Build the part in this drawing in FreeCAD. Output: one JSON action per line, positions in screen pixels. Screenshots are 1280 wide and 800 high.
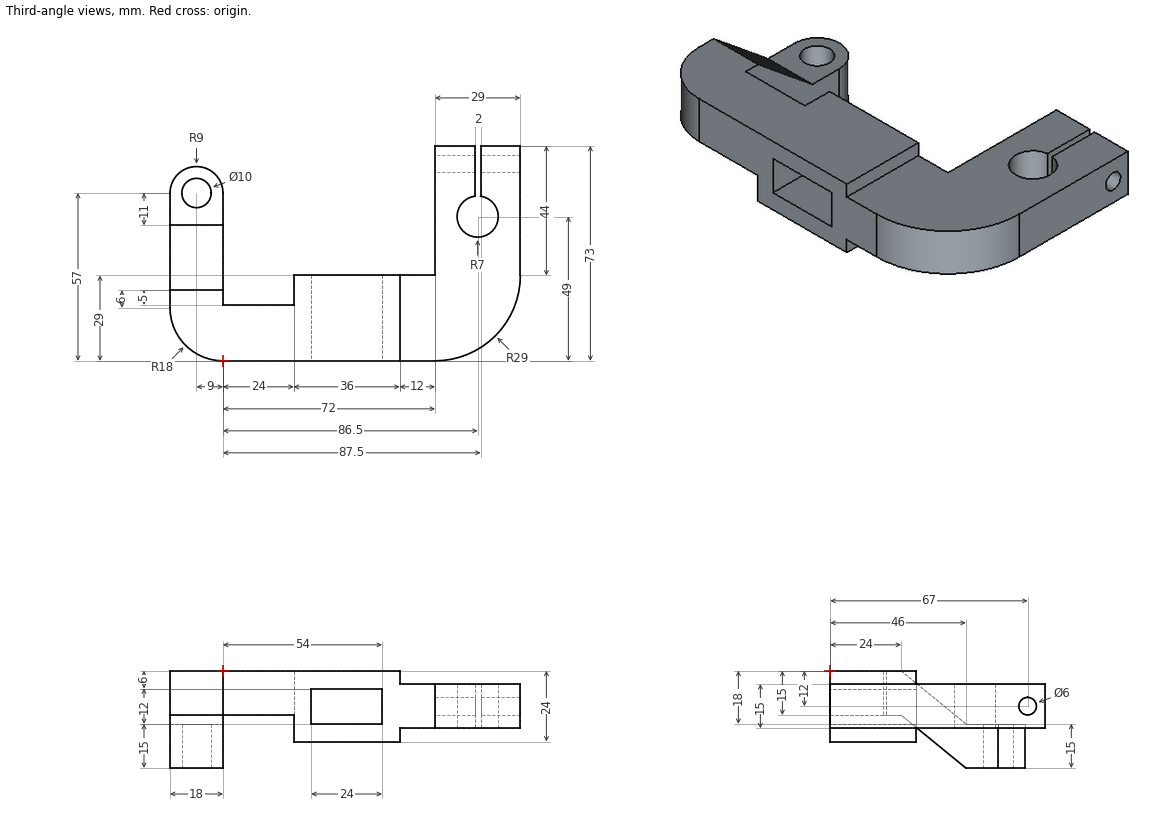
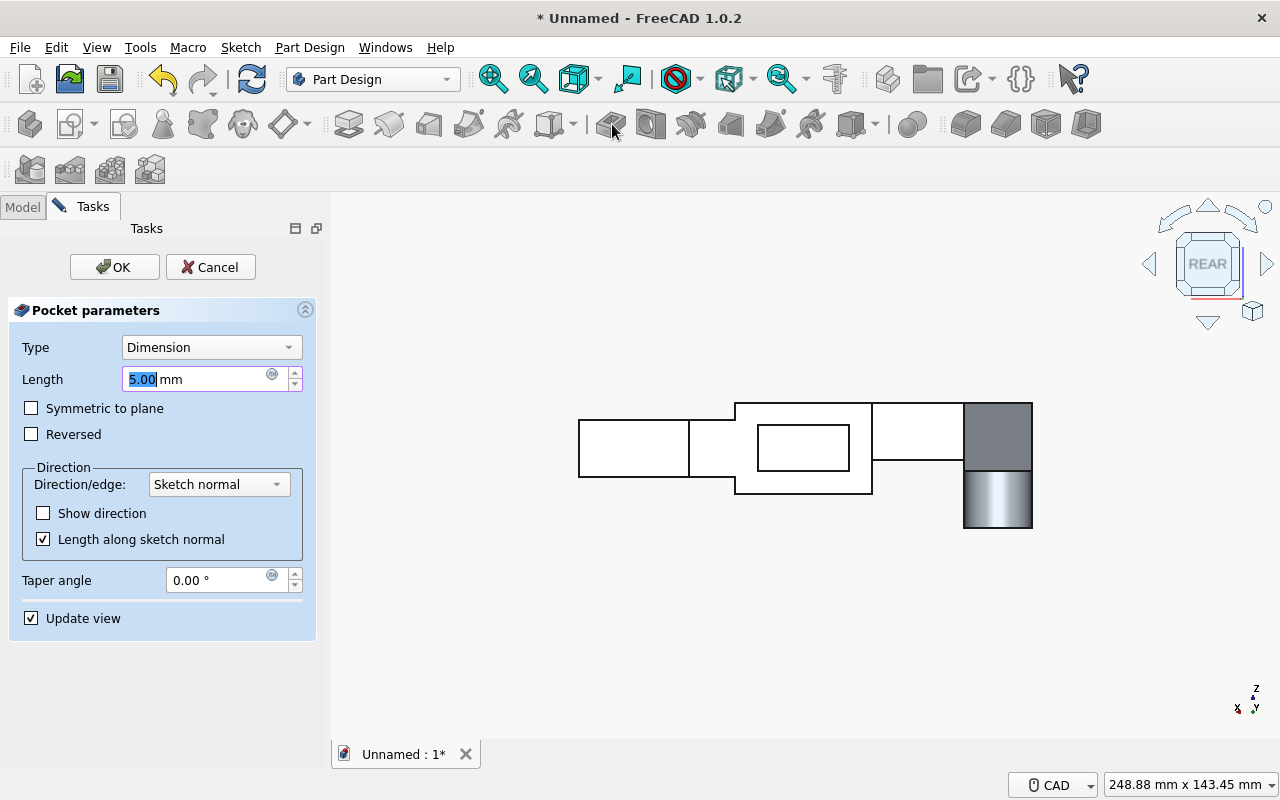
{"action": "left_click", "coordinate": [212, 348]}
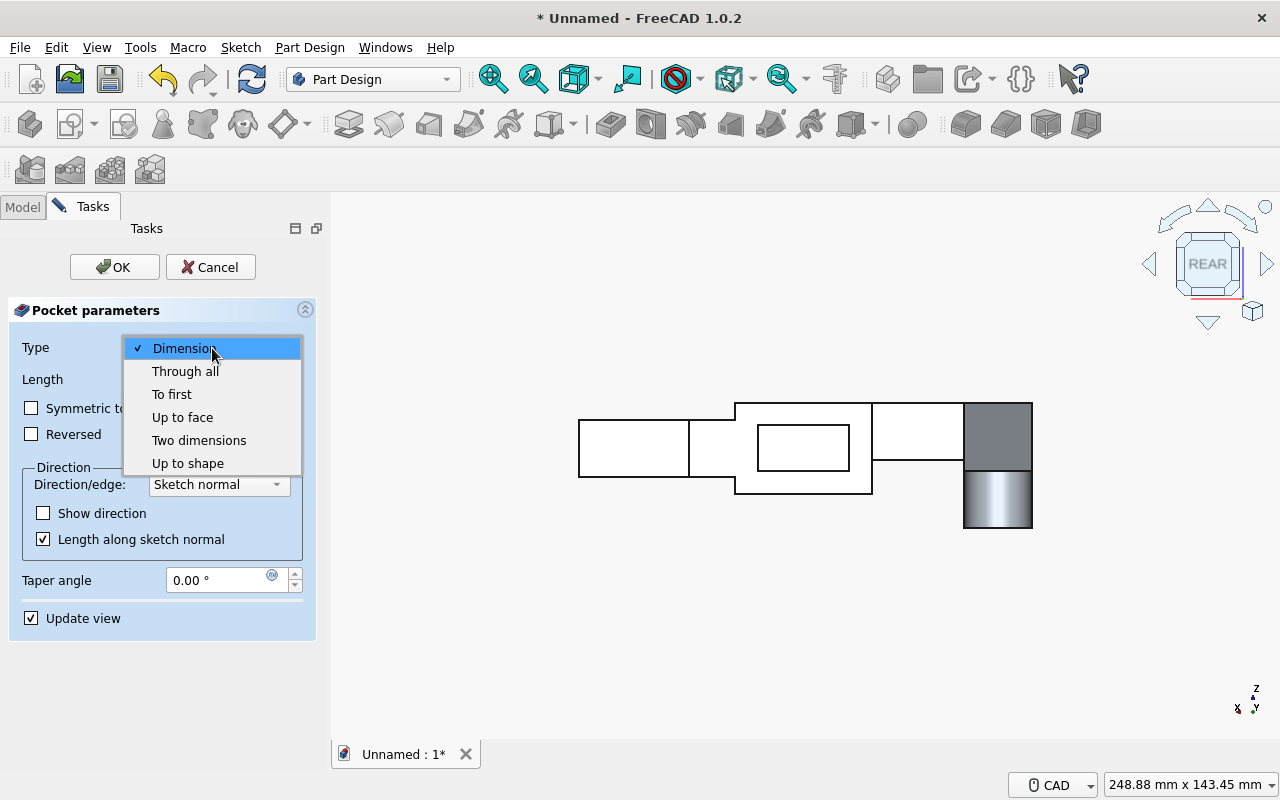
{"action": "left_click", "coordinate": [212, 372]}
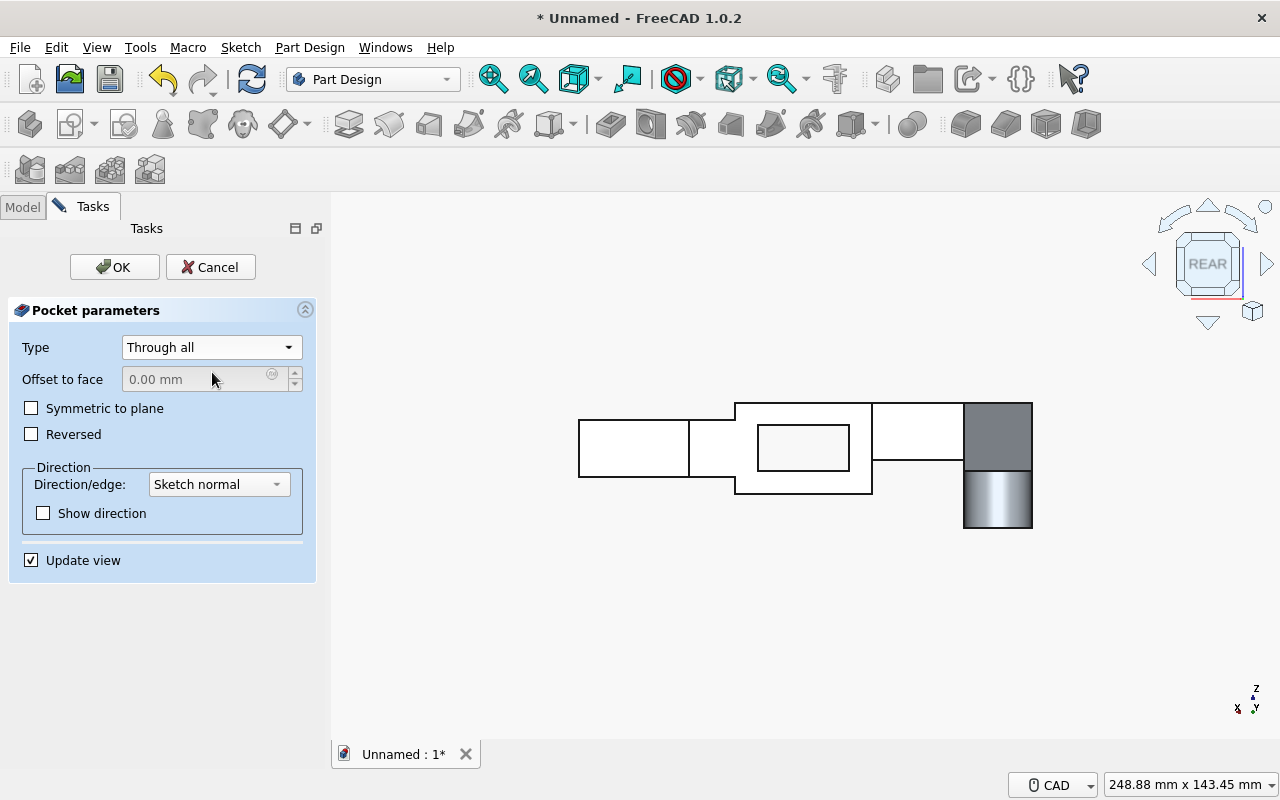
{"action": "left_click", "coordinate": [115, 267]}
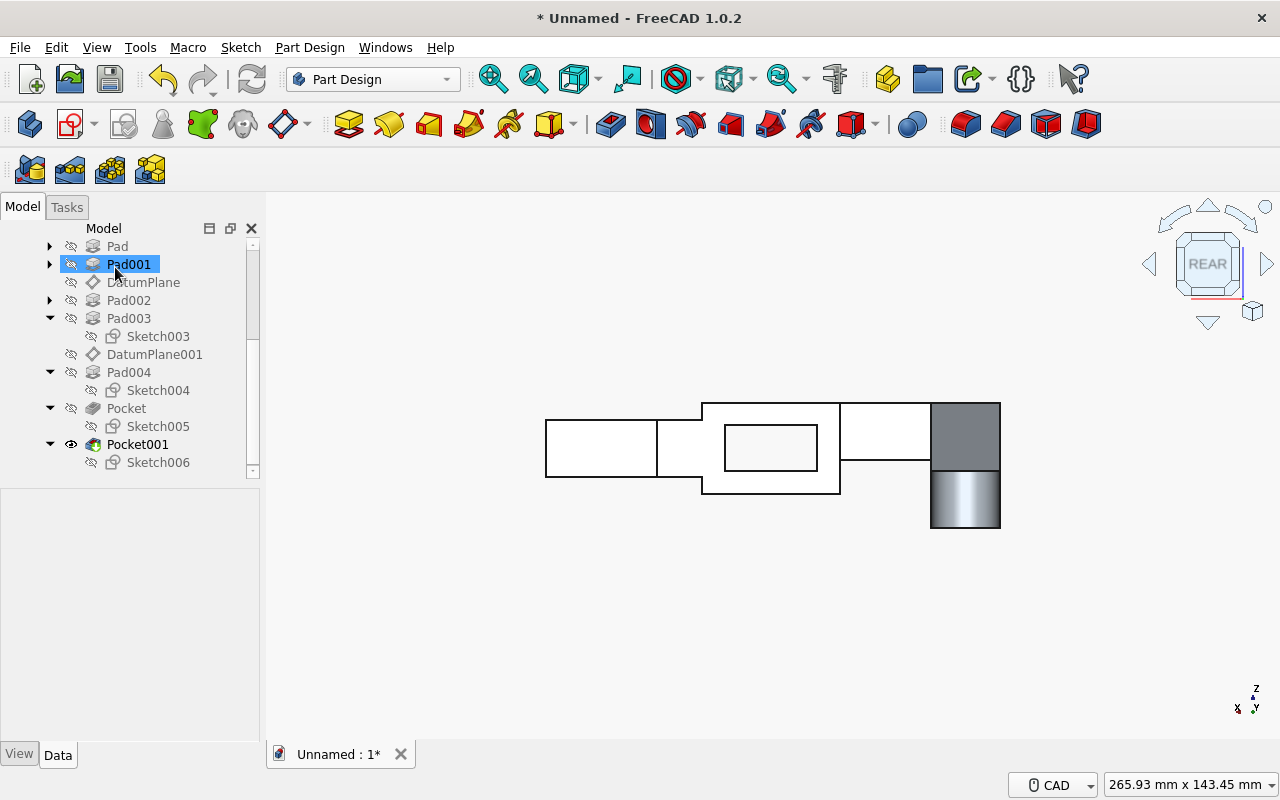
{"action": "key", "text": "v f"}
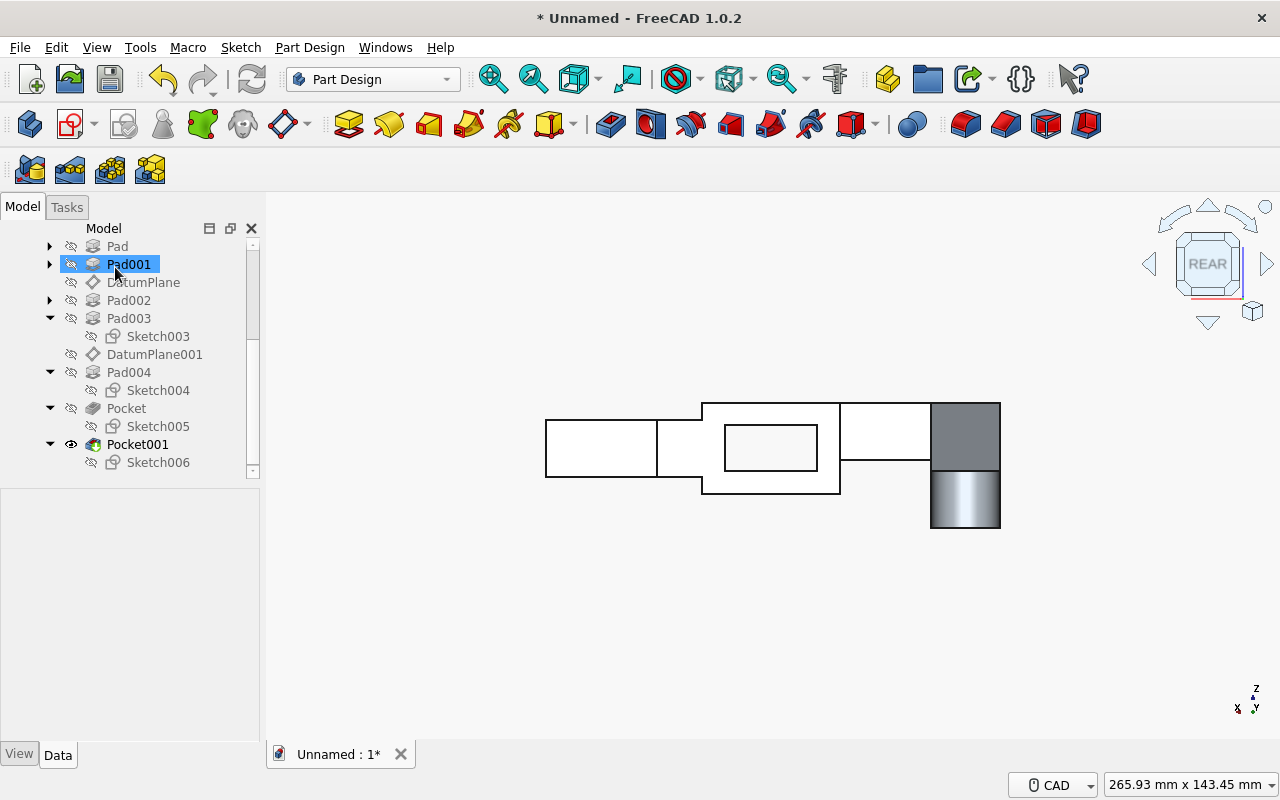
{"action": "key", "text": "0"}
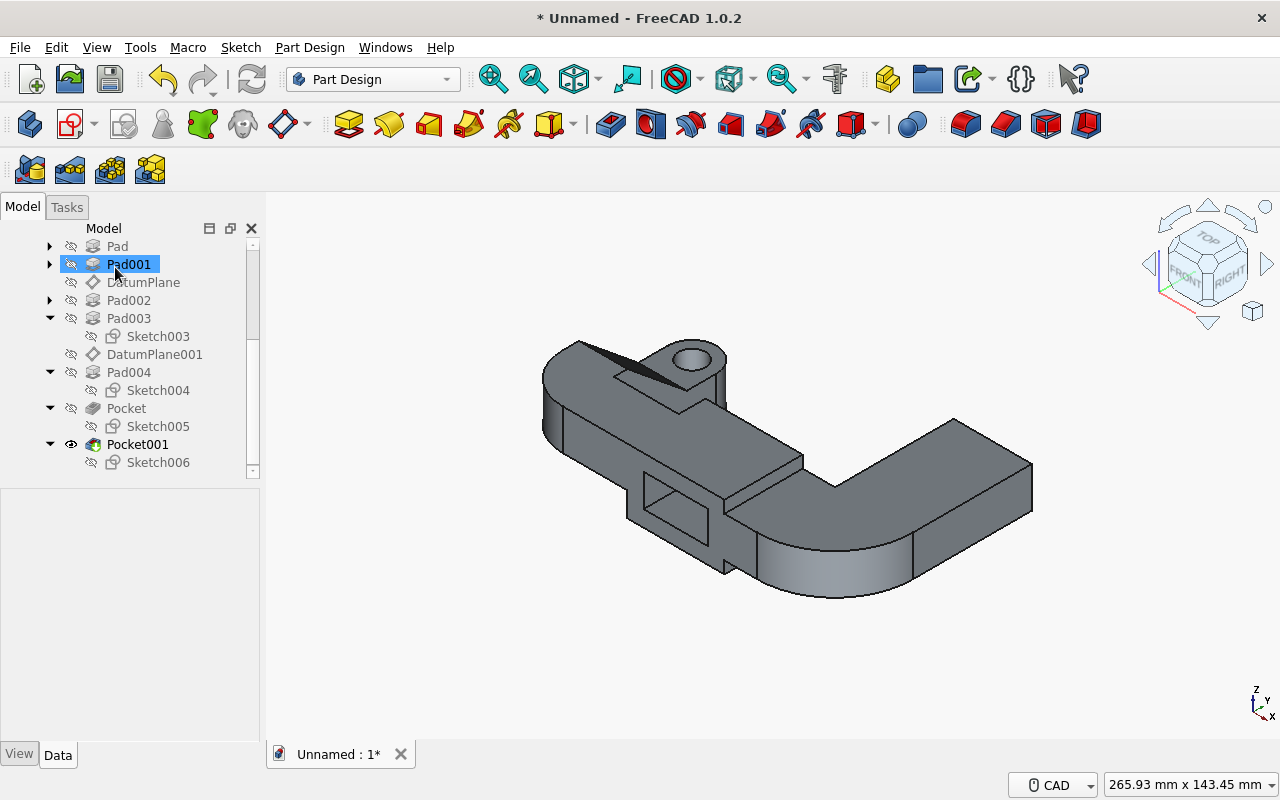
{"action": "left_click", "coordinate": [950, 464]}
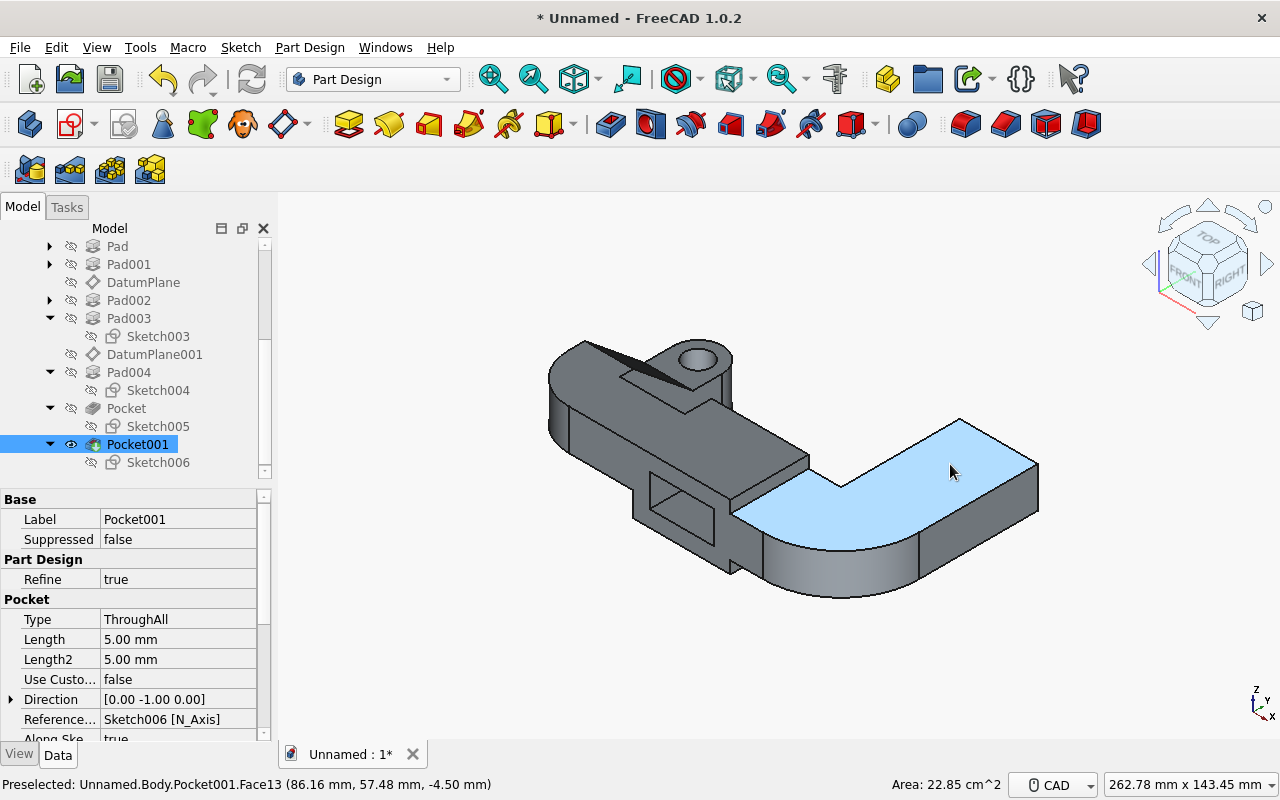
{"action": "left_click", "coordinate": [70, 124]}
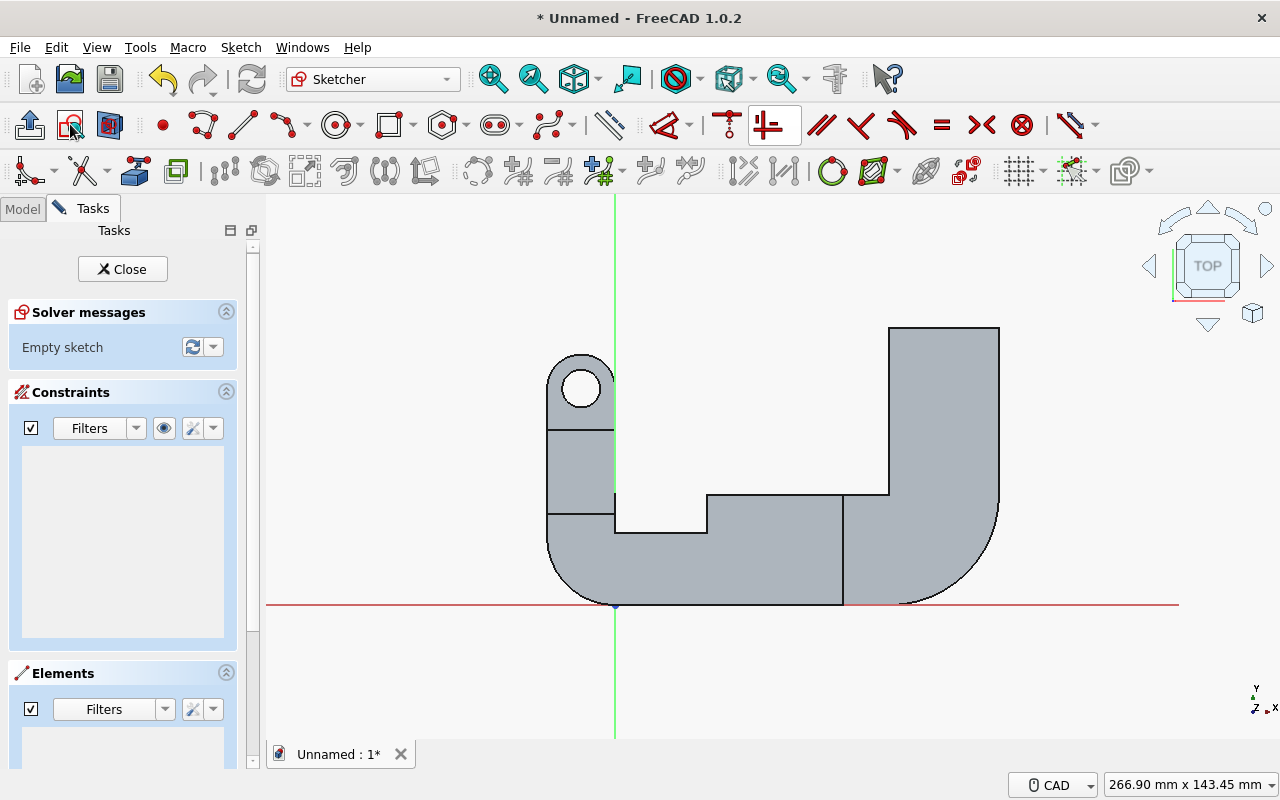
{"action": "left_click", "coordinate": [110, 126]}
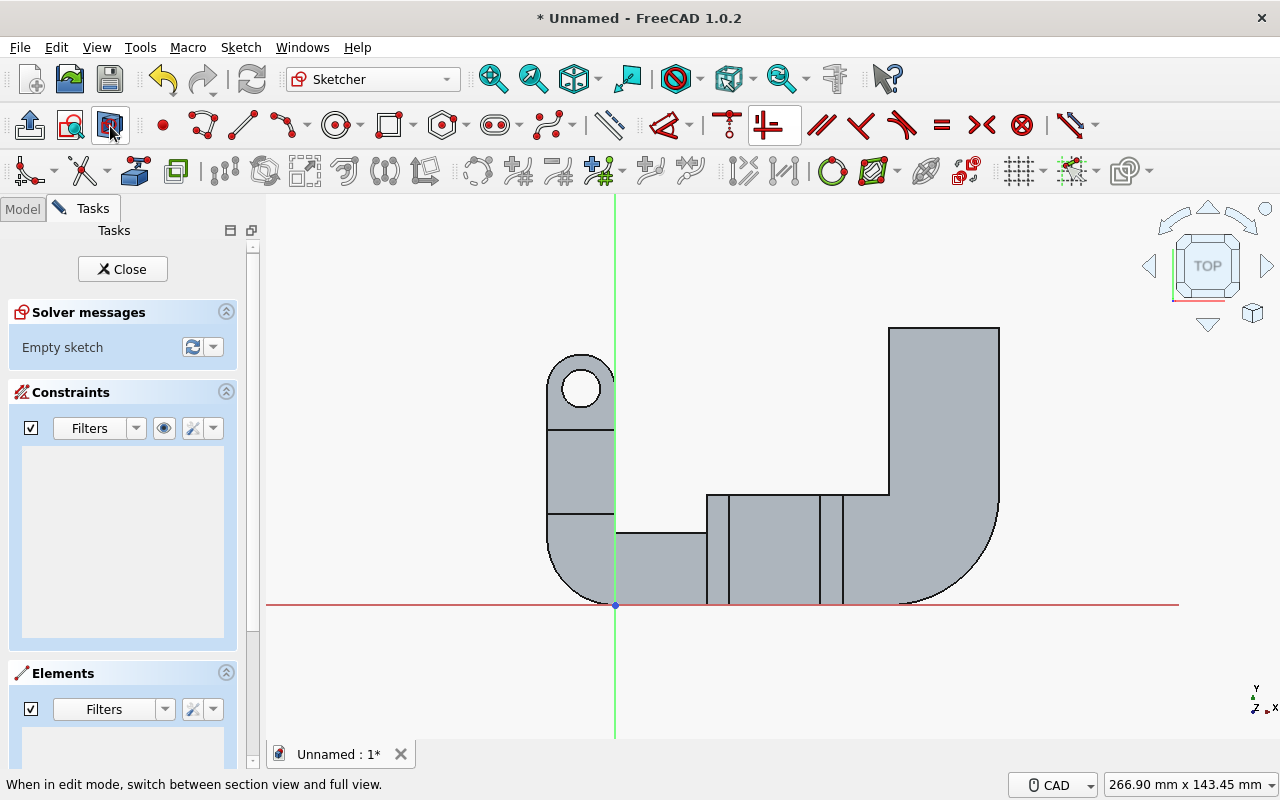
{"action": "scroll", "coordinate": [1083, 340], "scroll_direction": "up", "scroll_amount": 5}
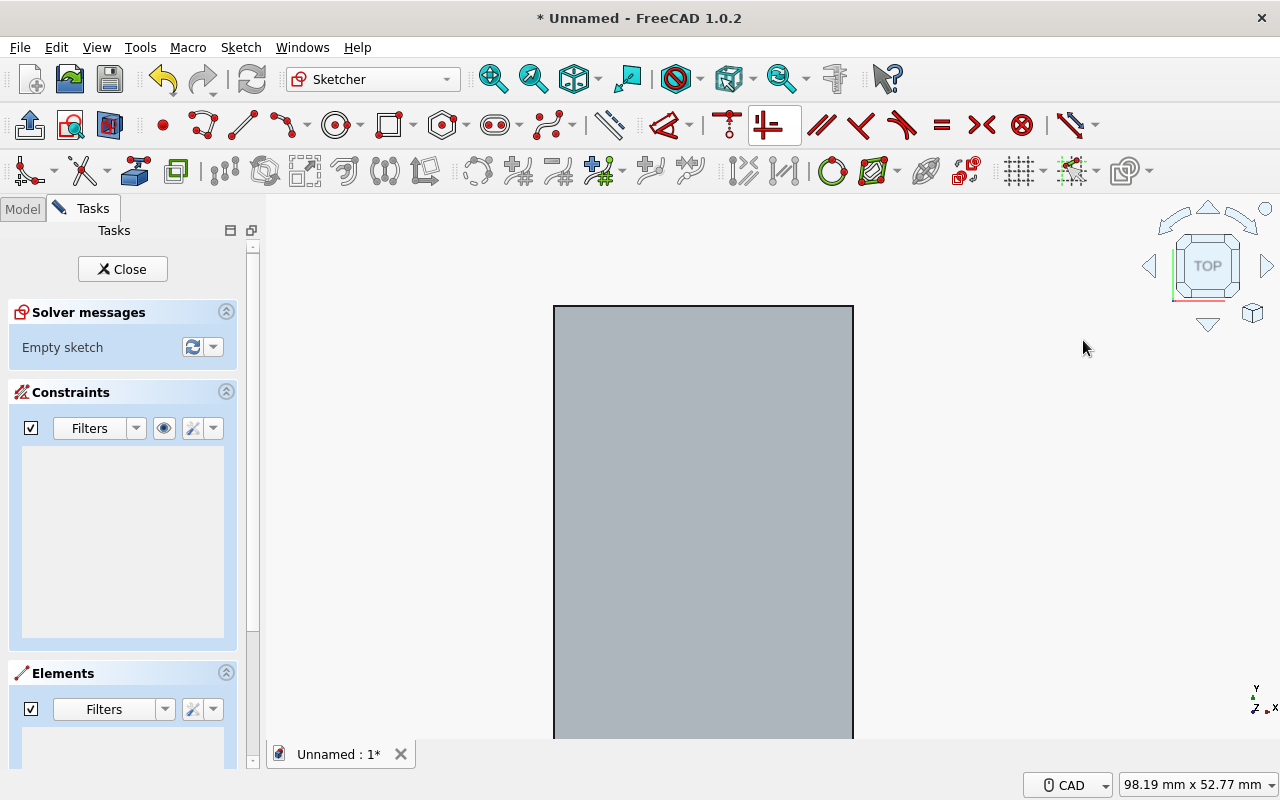
{"action": "key", "text": "g m"}